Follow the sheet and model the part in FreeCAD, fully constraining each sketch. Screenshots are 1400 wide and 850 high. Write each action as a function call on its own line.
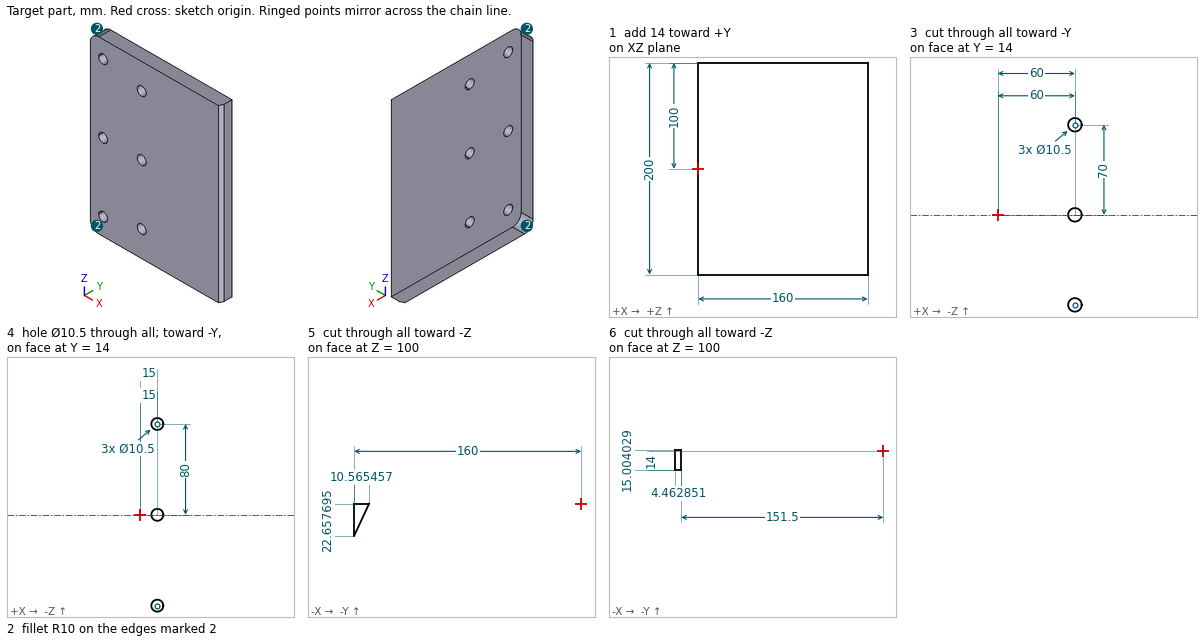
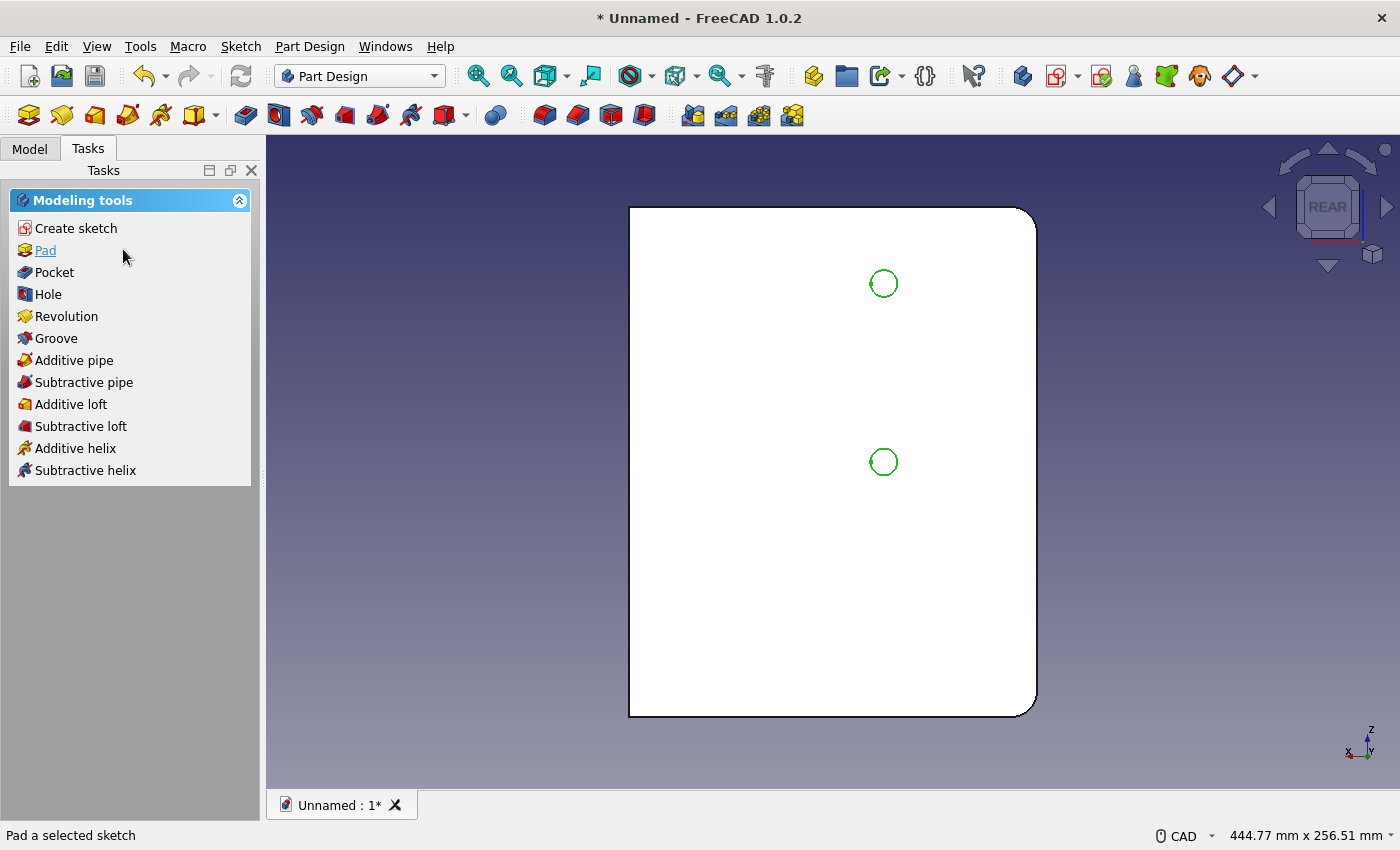
click(246, 116)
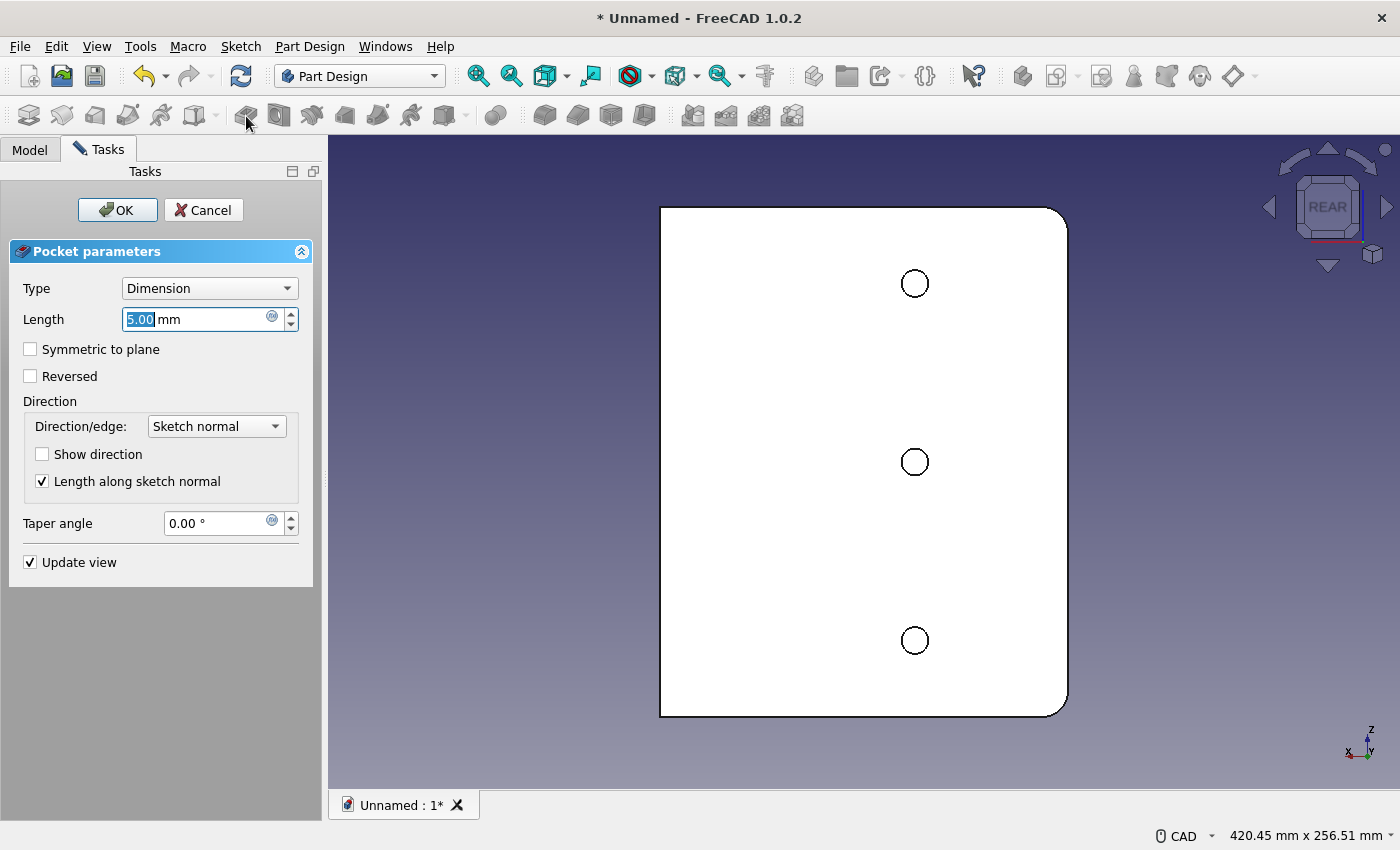
click(210, 288)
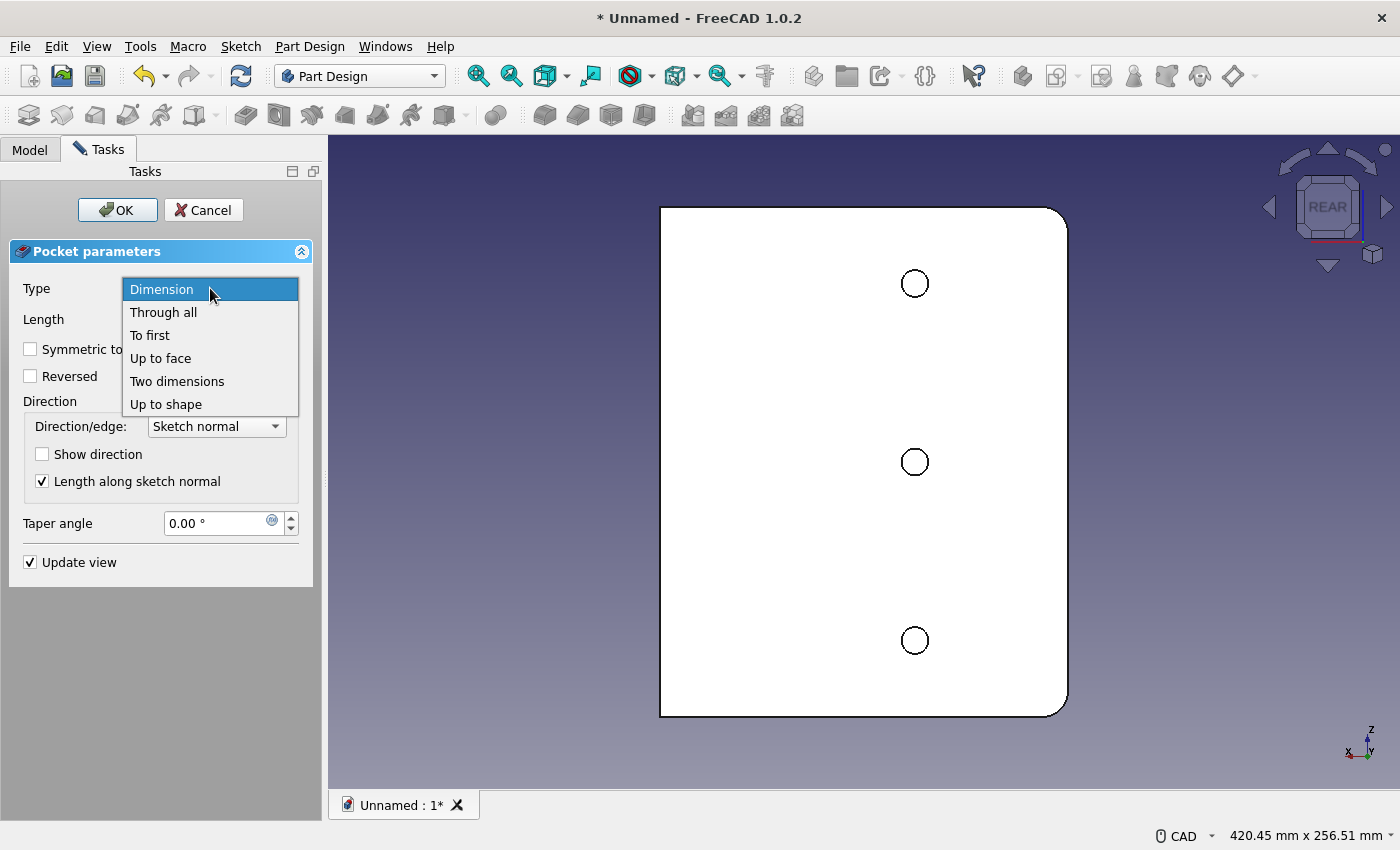
click(208, 312)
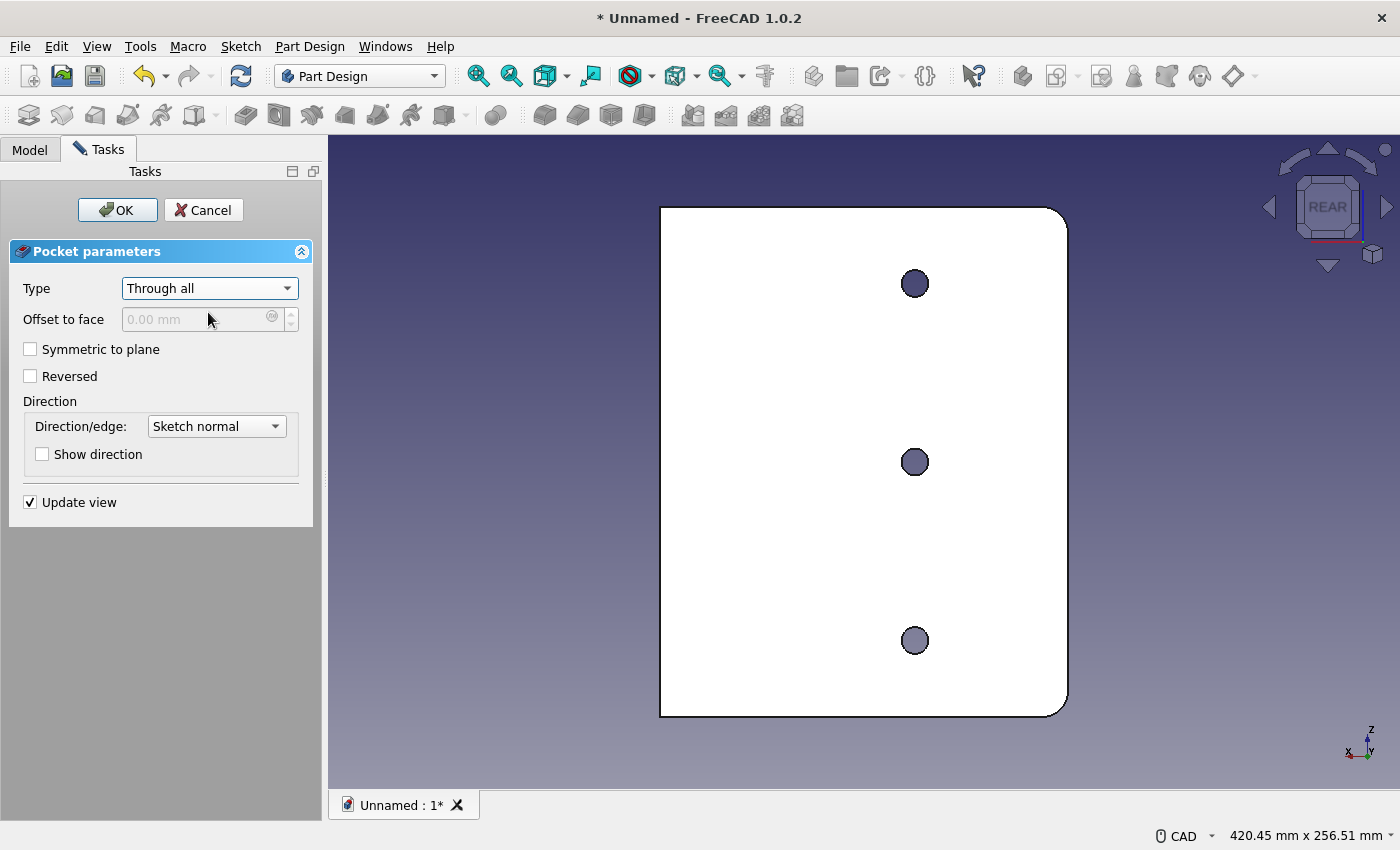
click(118, 210)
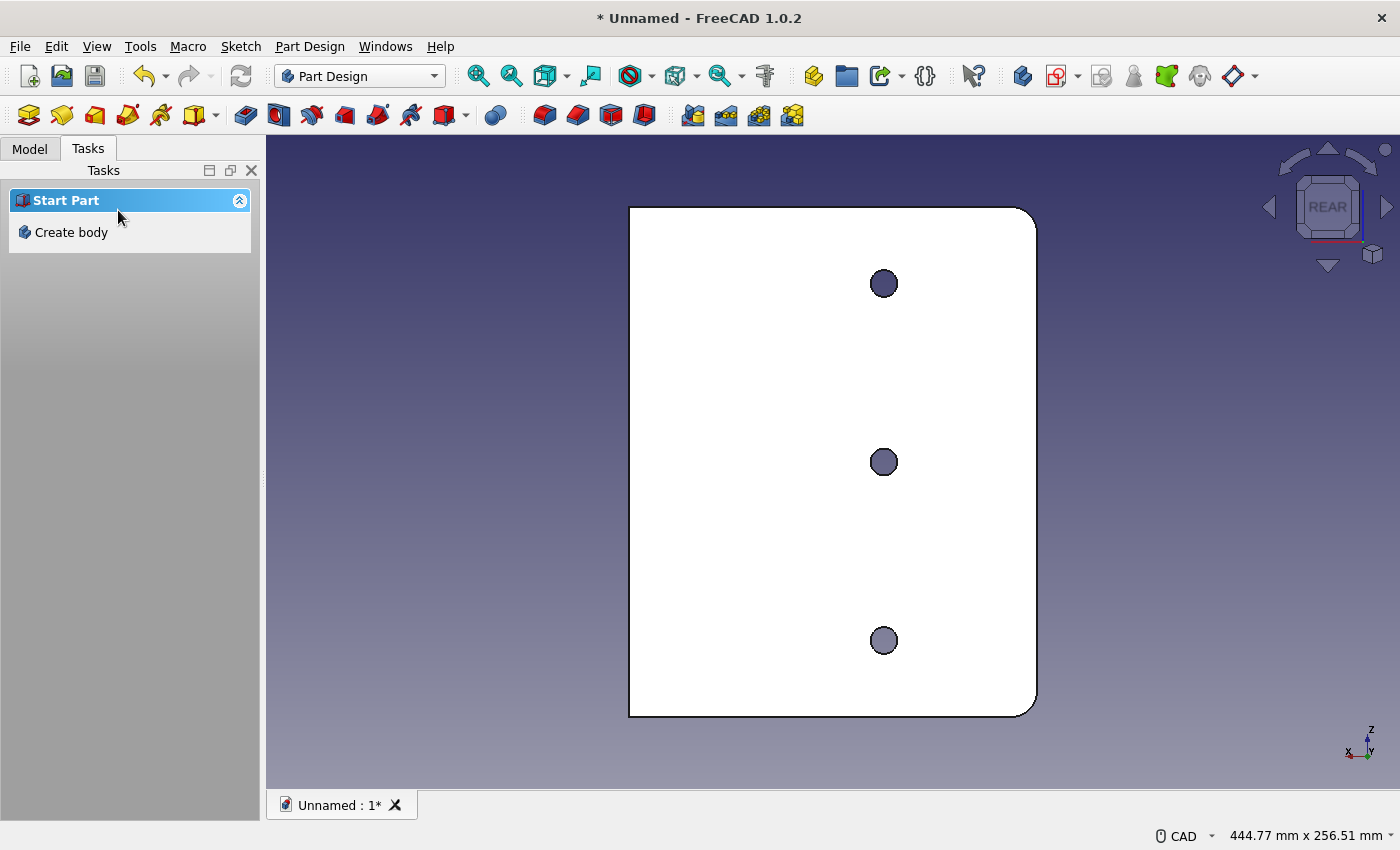
click(775, 388)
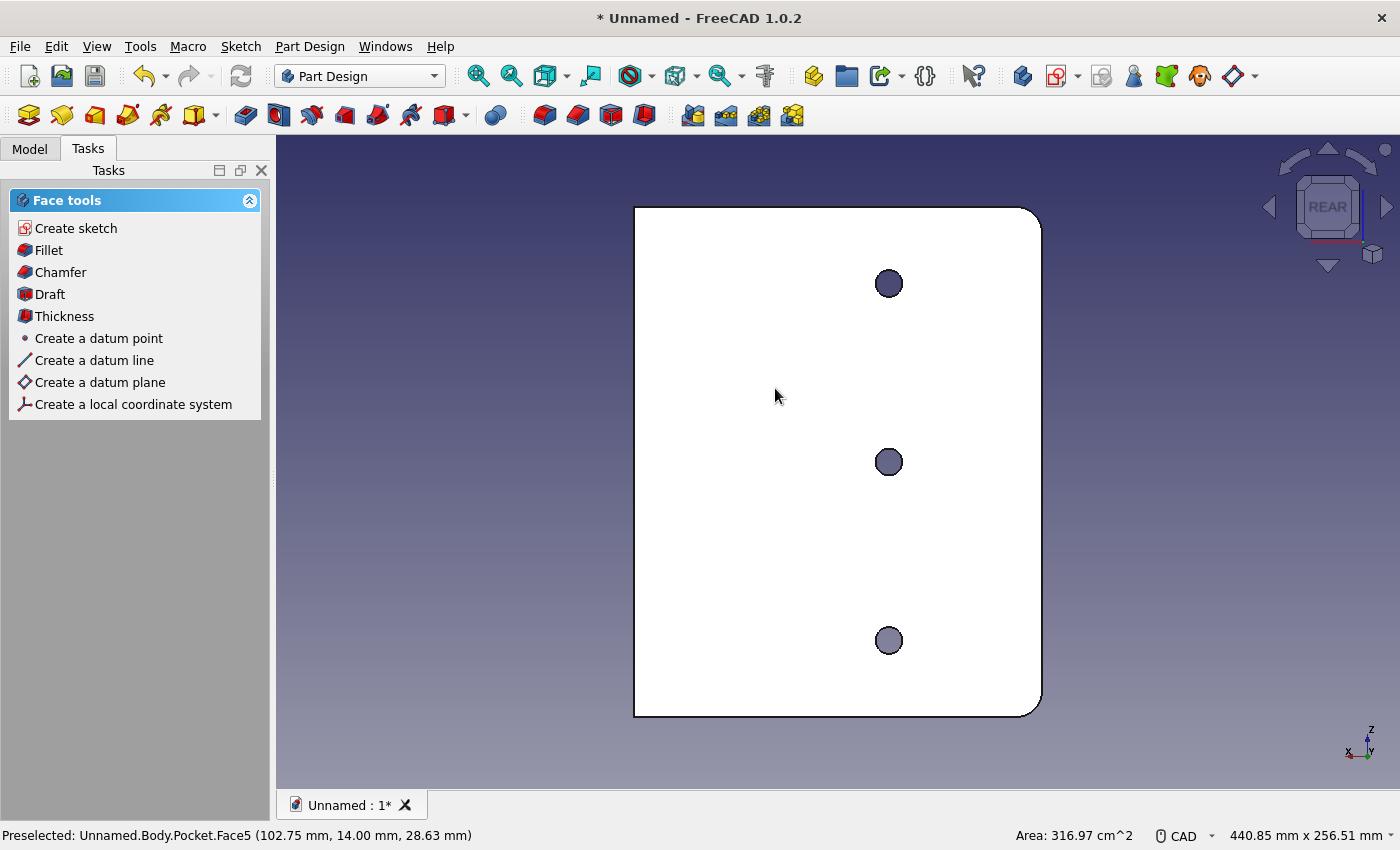
click(1056, 76)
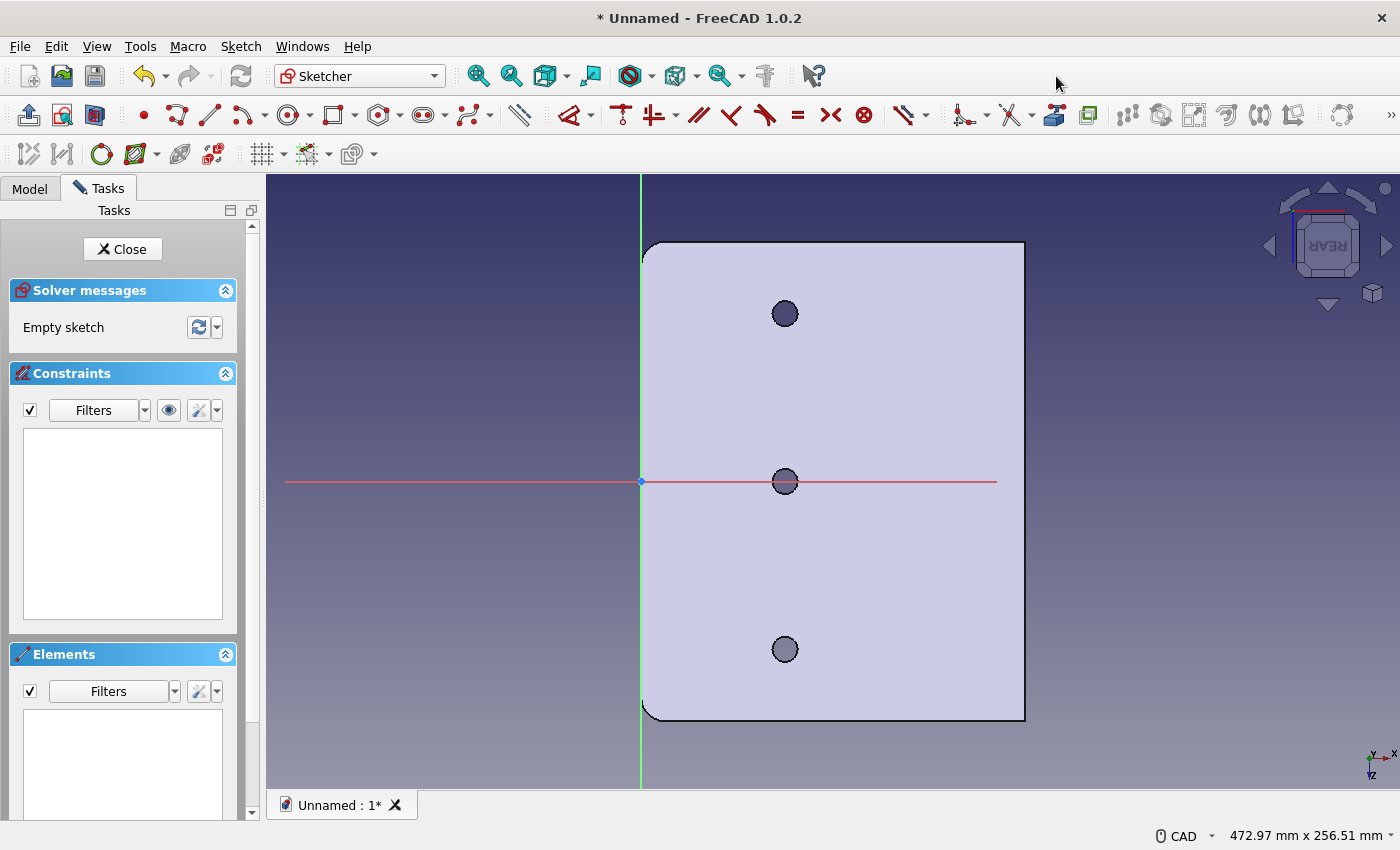
key(g)
key(c)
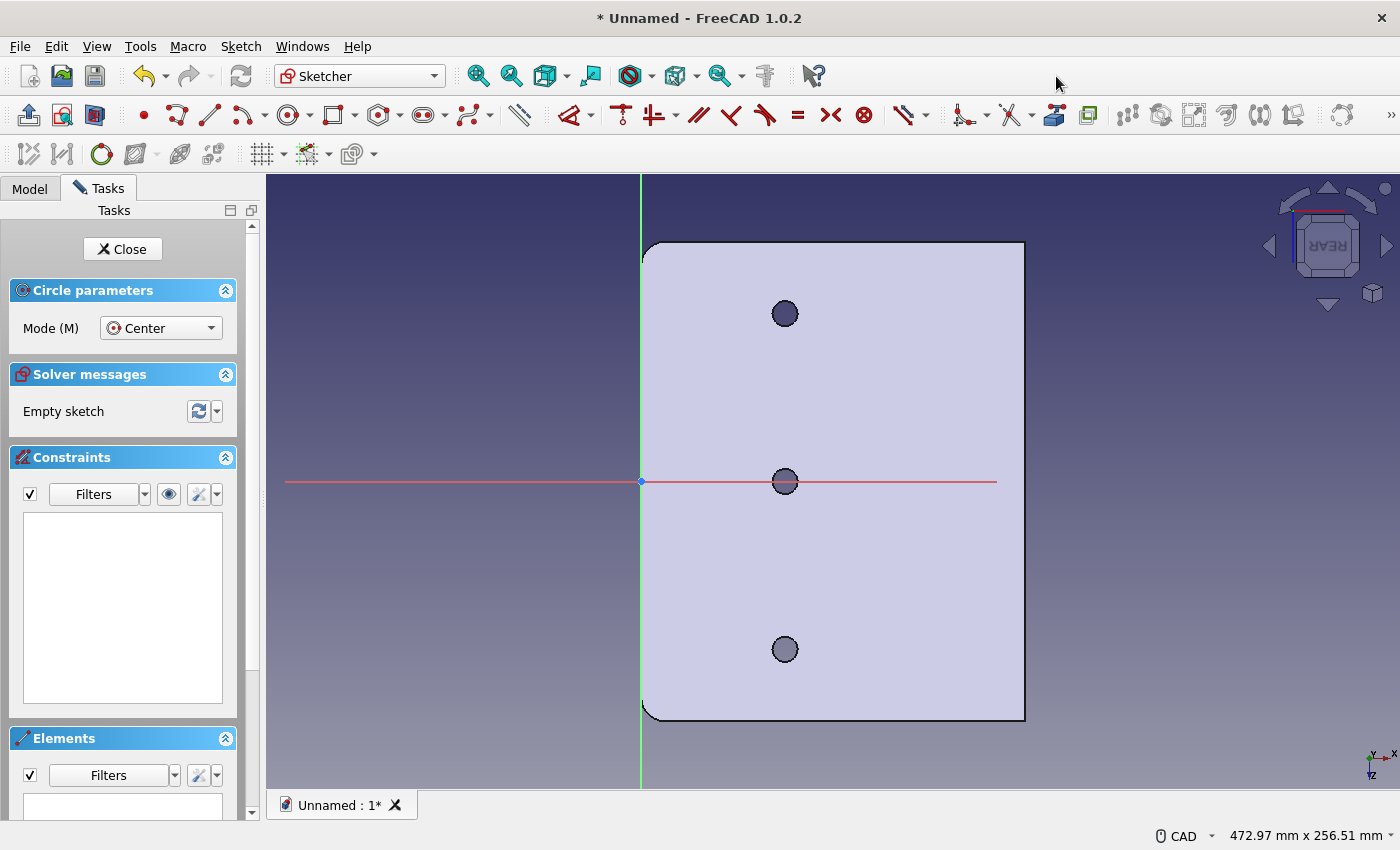
scroll(677, 290, up, 3)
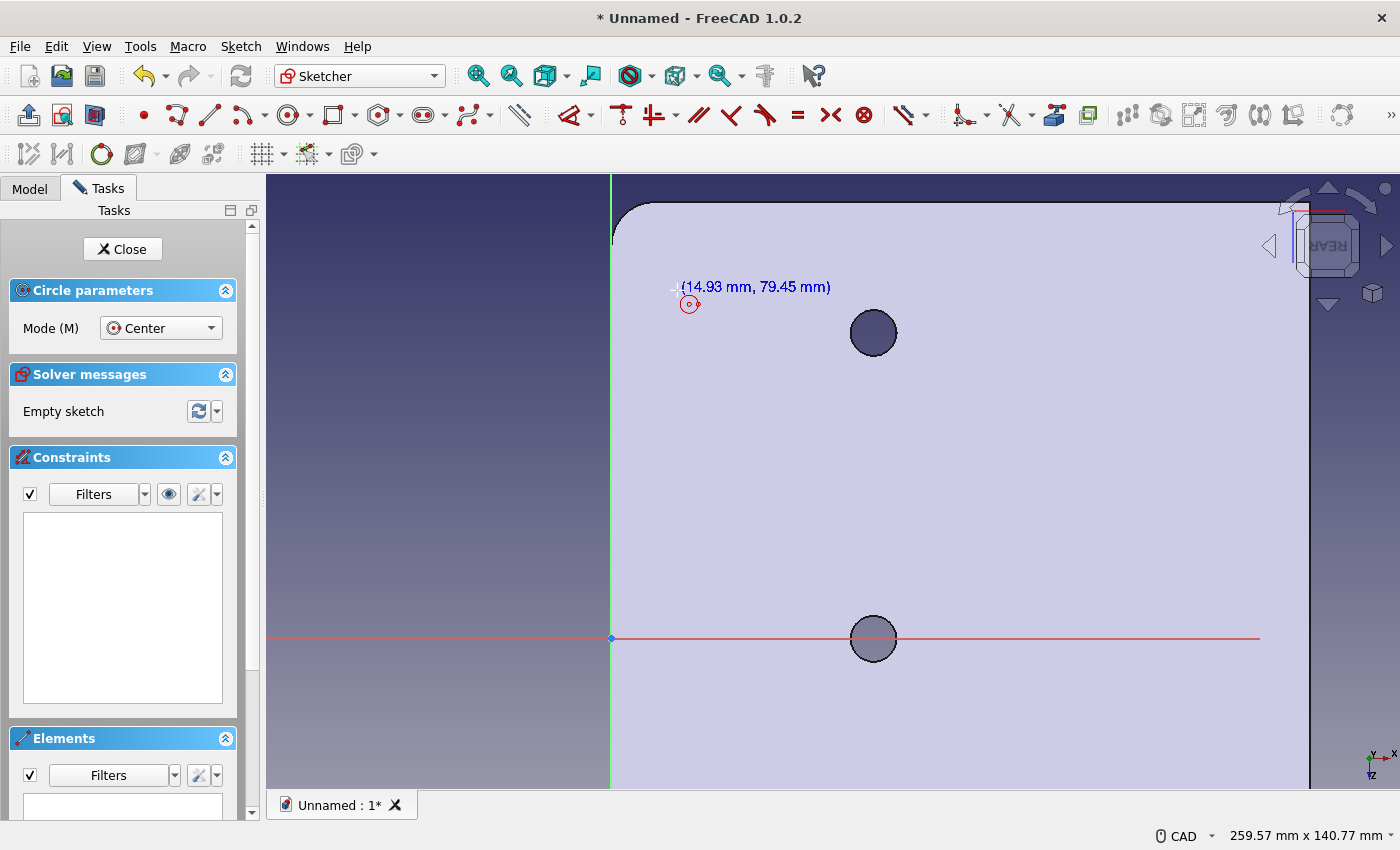
click(677, 289)
click(693, 273)